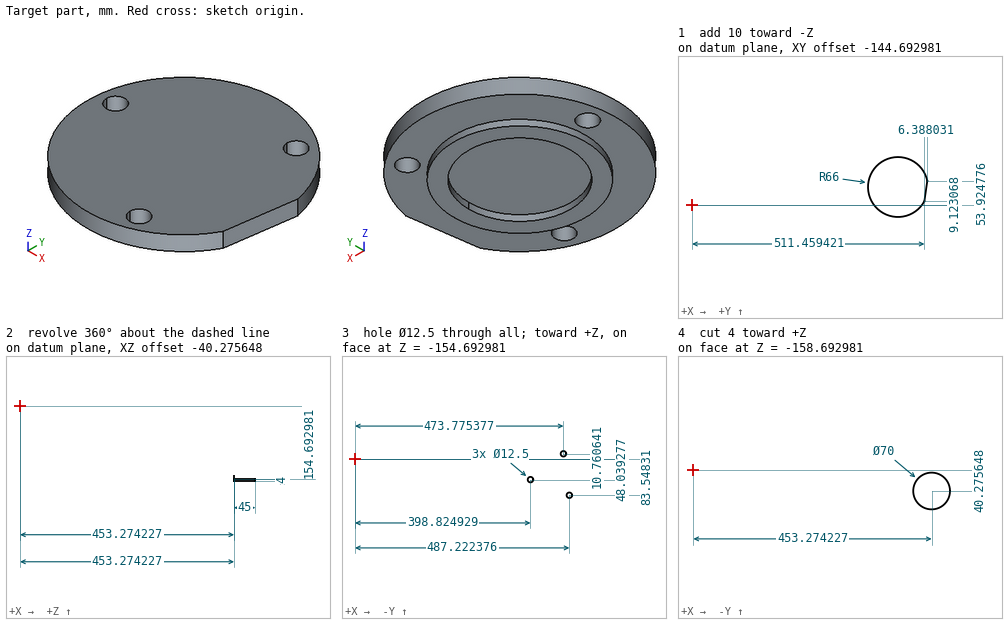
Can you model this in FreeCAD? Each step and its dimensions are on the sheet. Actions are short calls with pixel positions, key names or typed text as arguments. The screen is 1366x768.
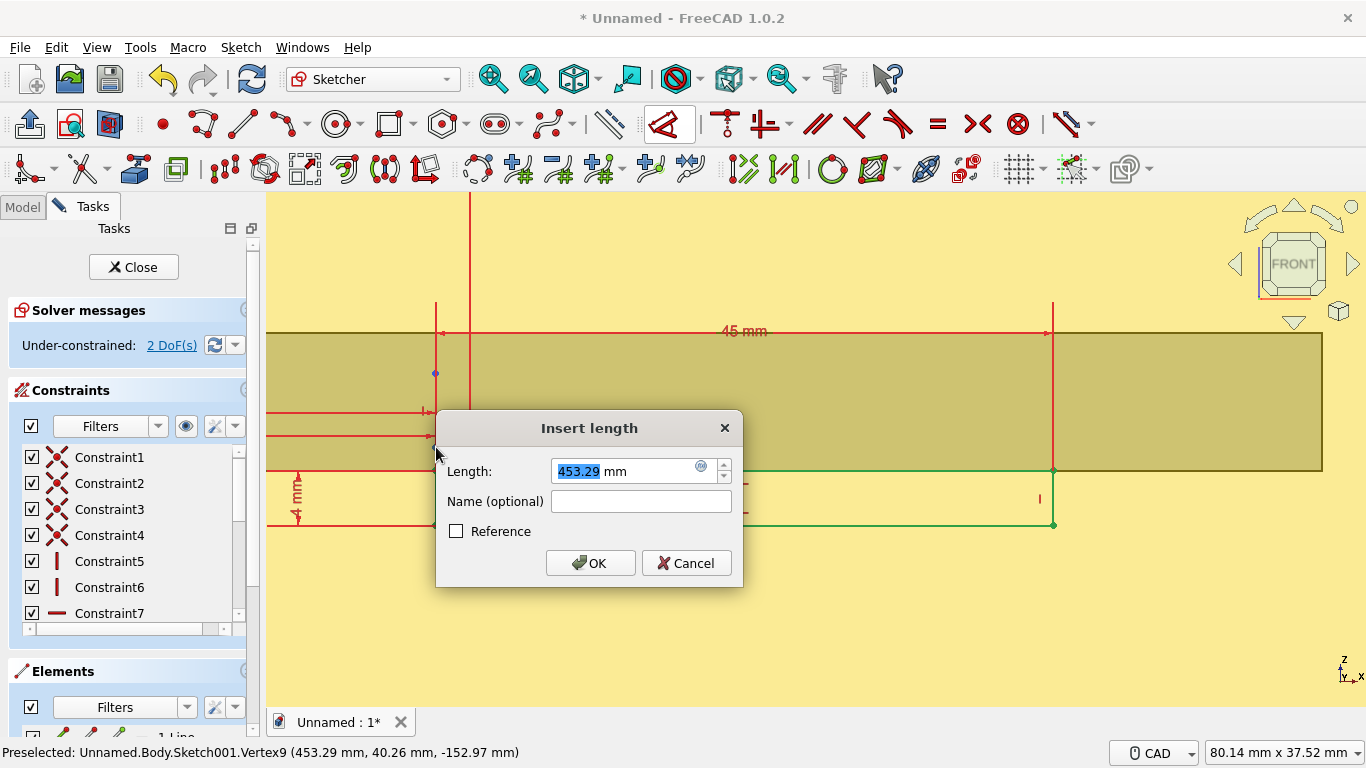
text(453.274227)
key(Return)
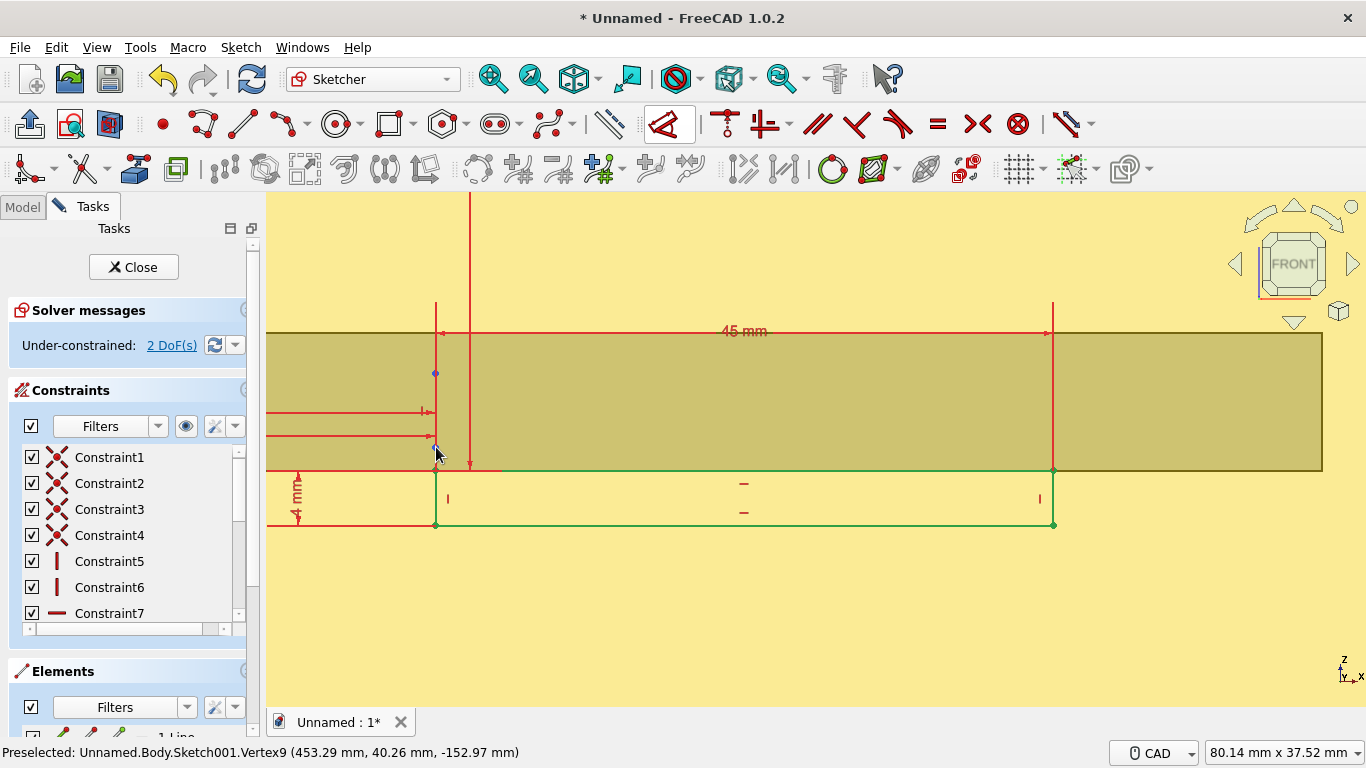
click(134, 267)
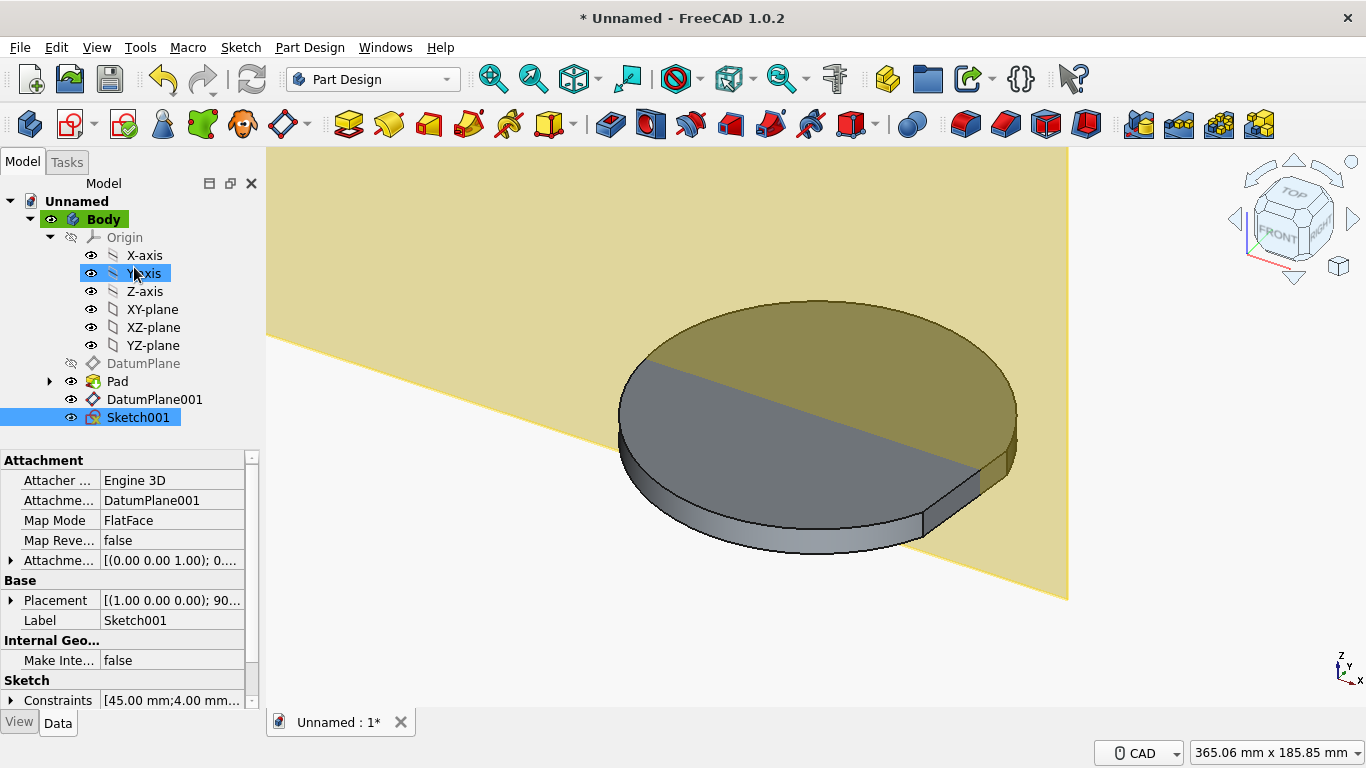
click(390, 124)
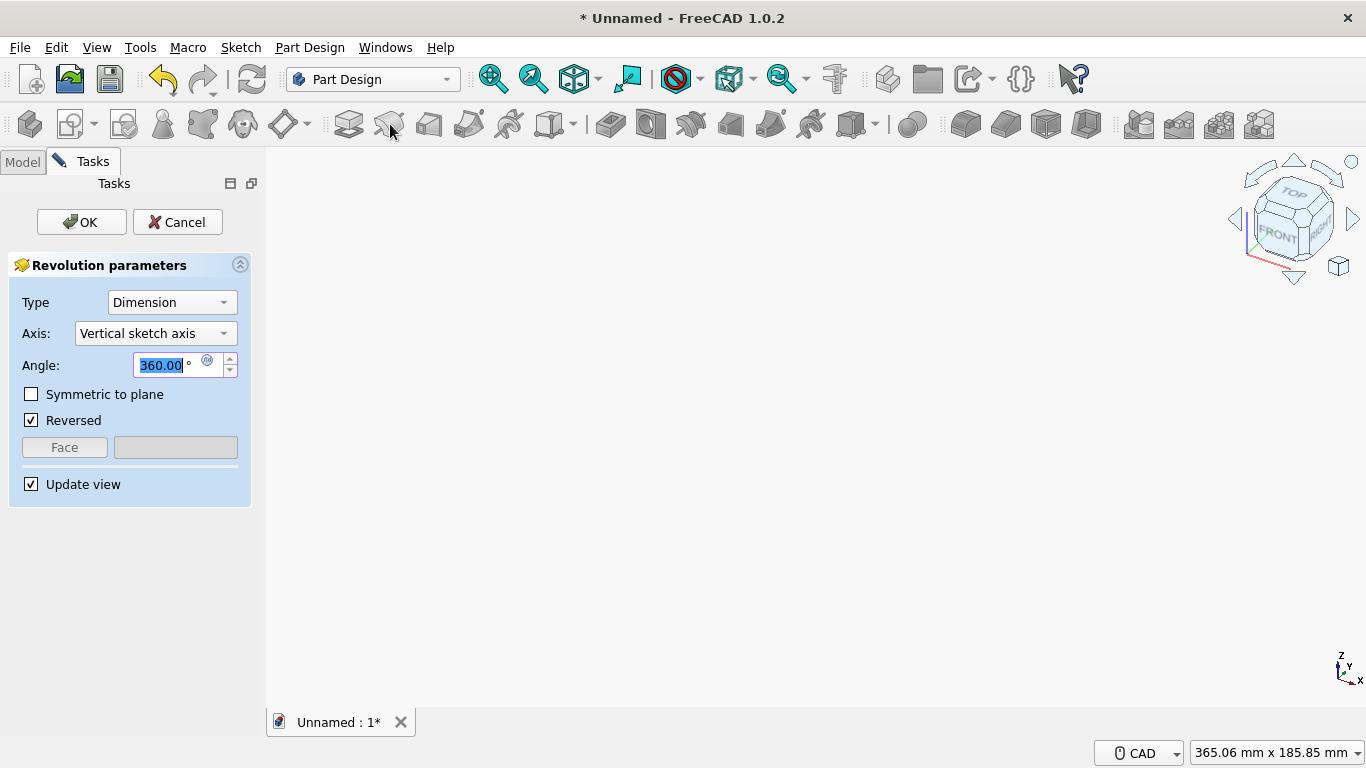
click(156, 334)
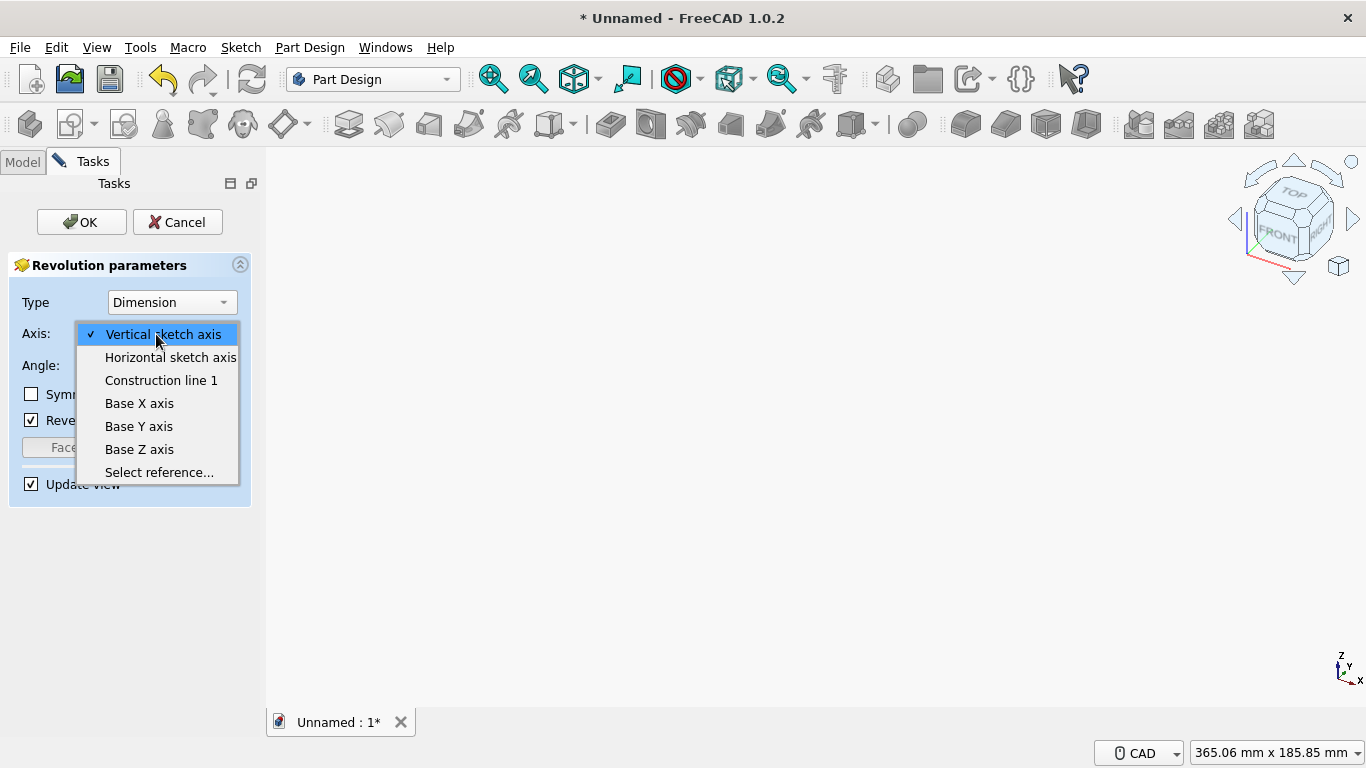
click(156, 380)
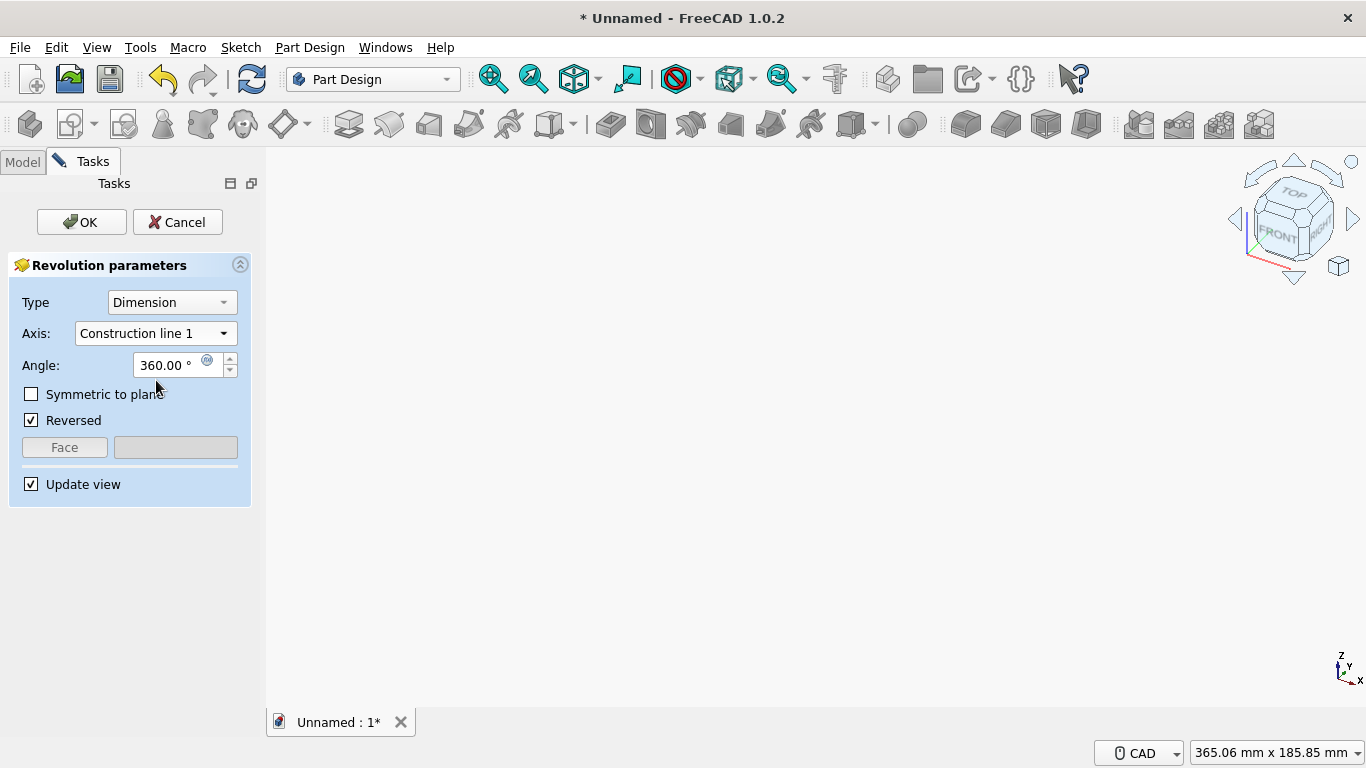
click(82, 222)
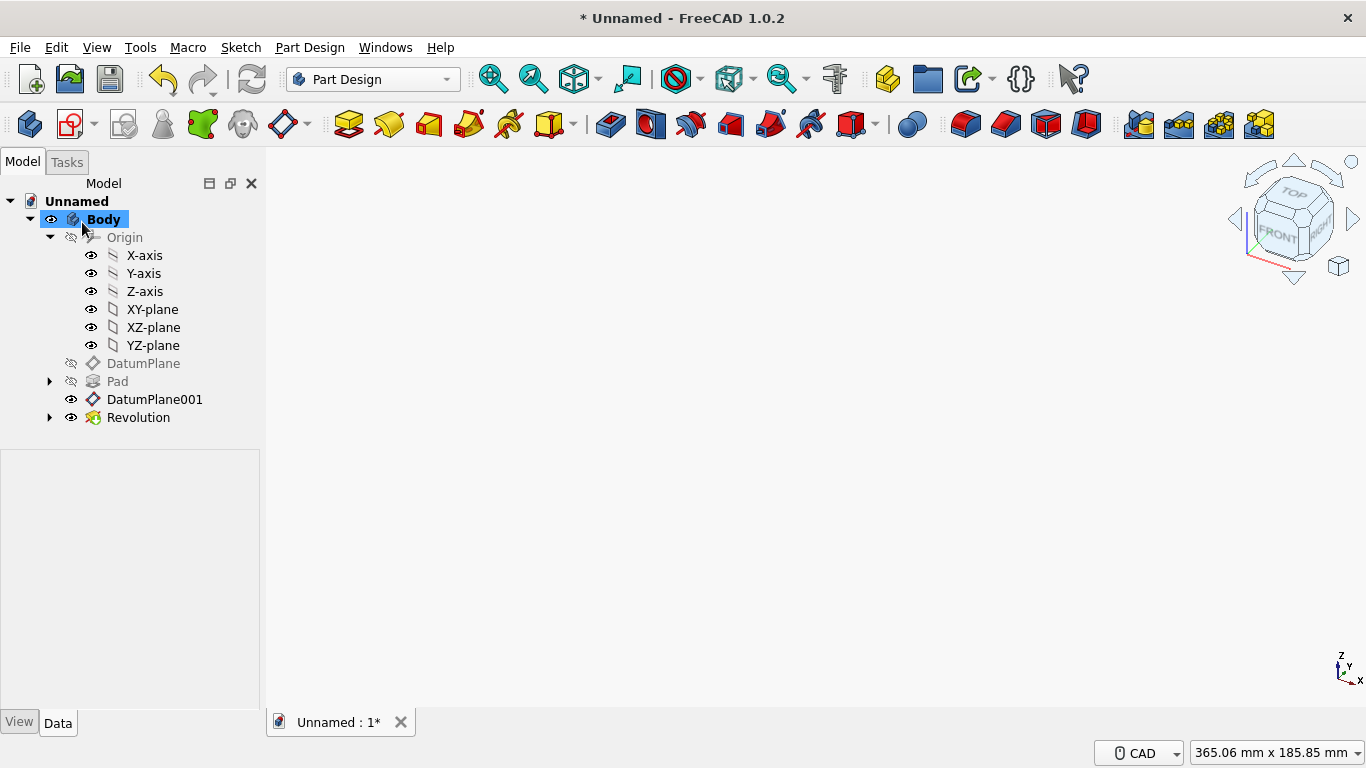
click(116, 399)
key(space)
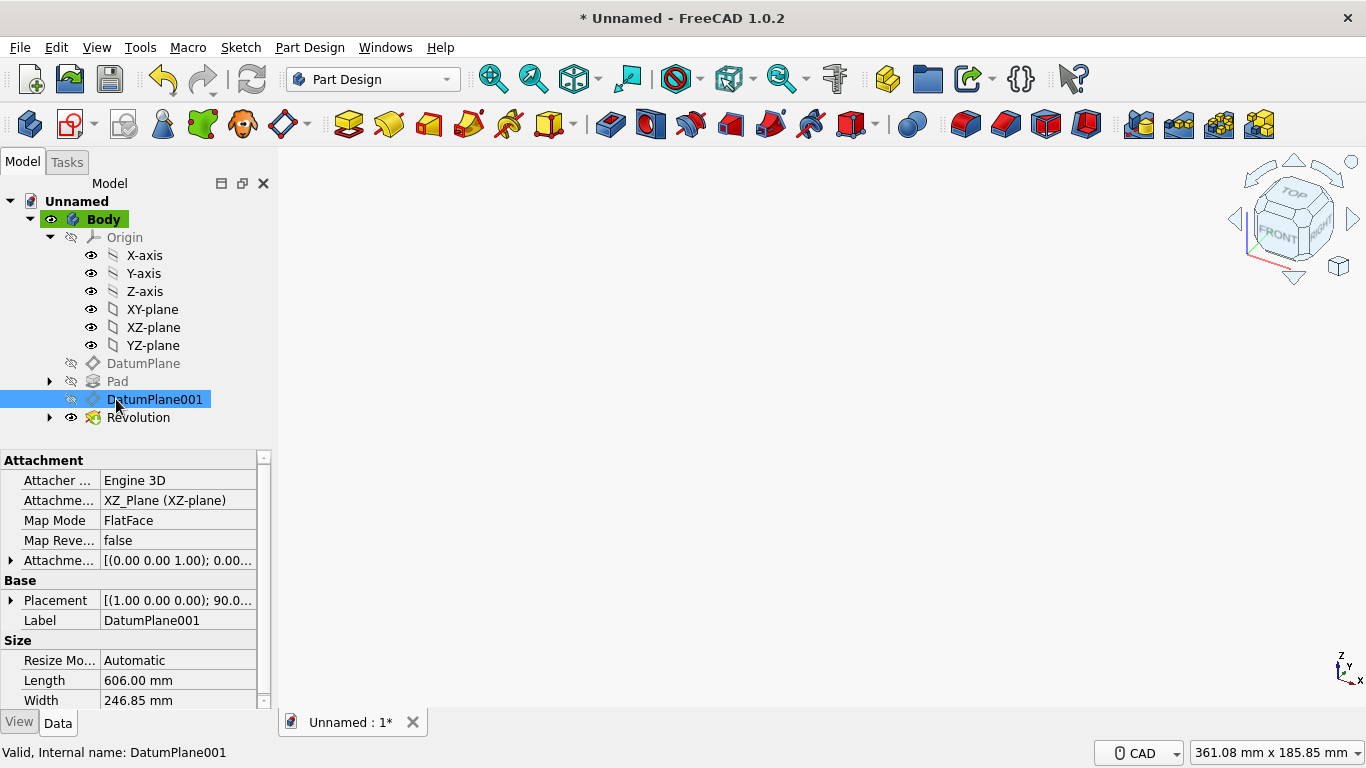
key(v)
key(f)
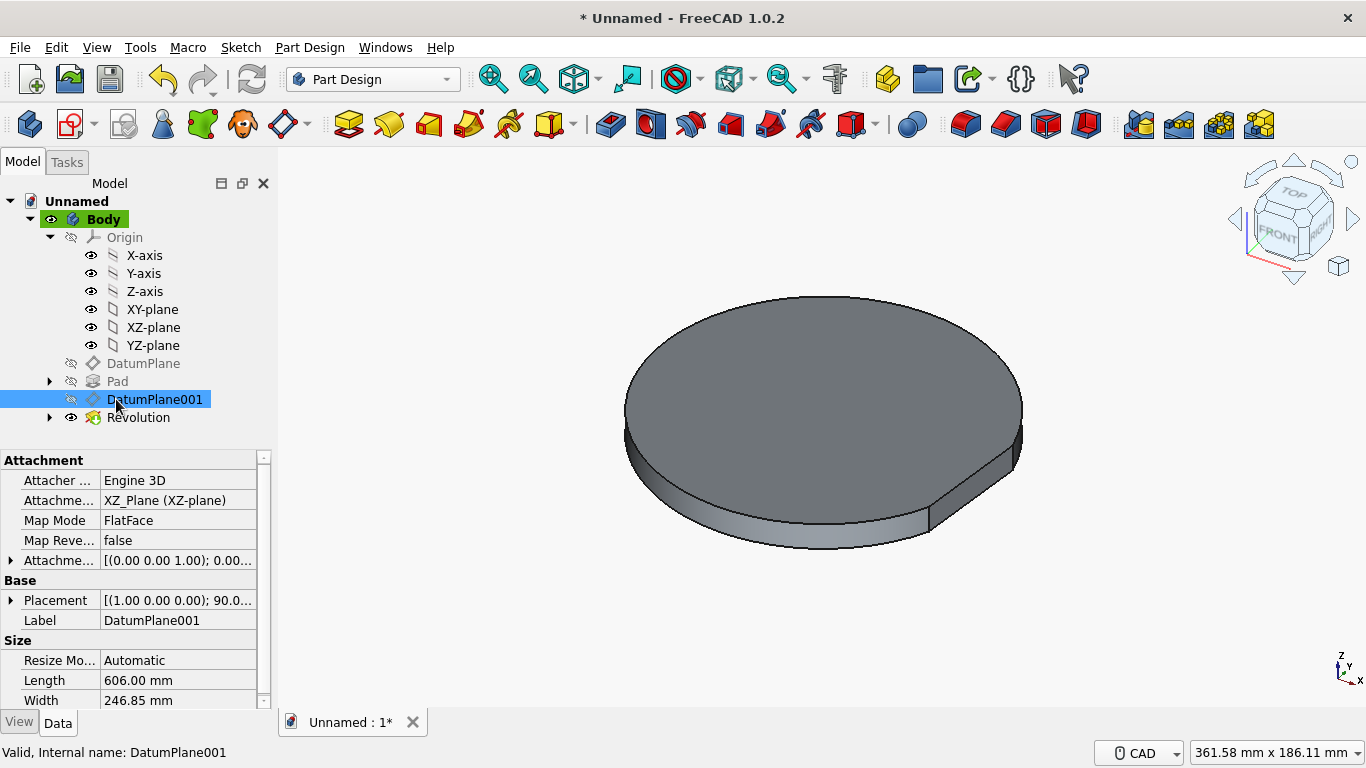
key(5)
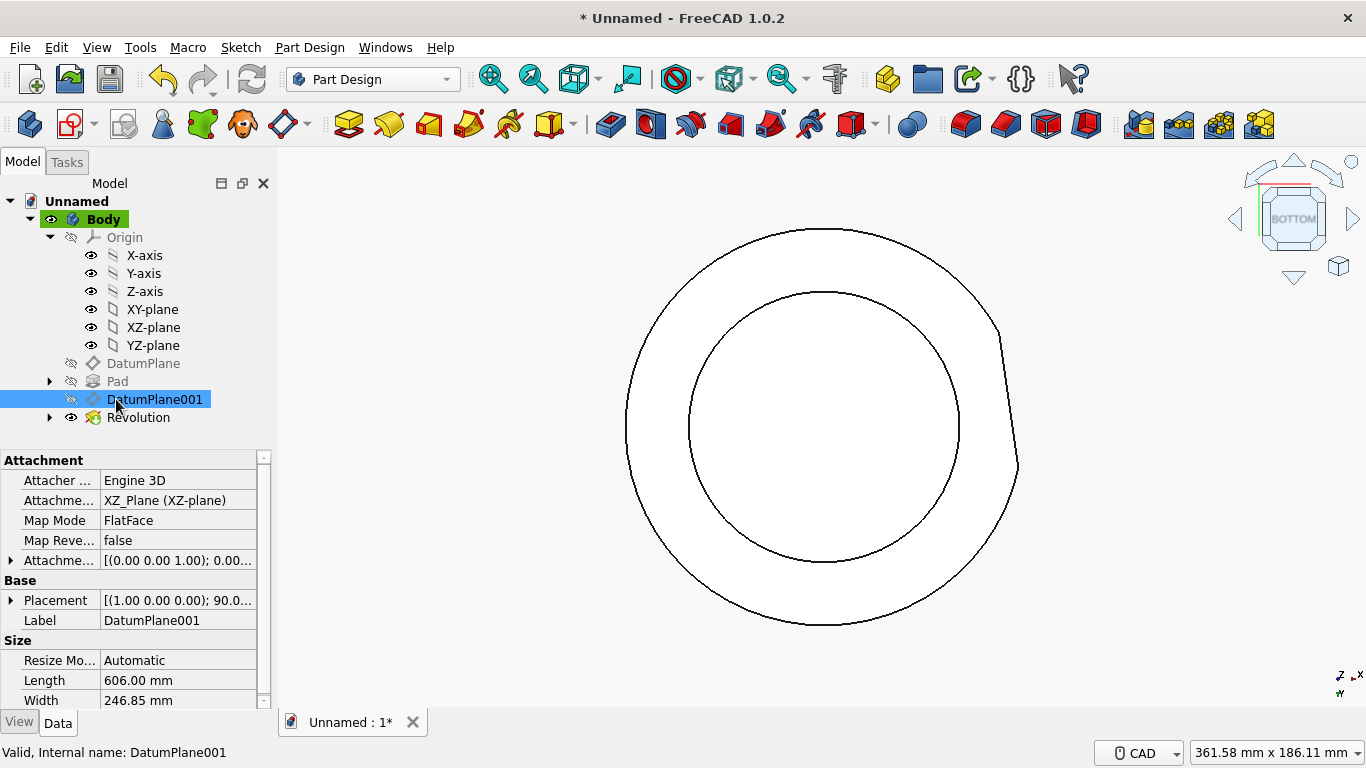
click(822, 596)